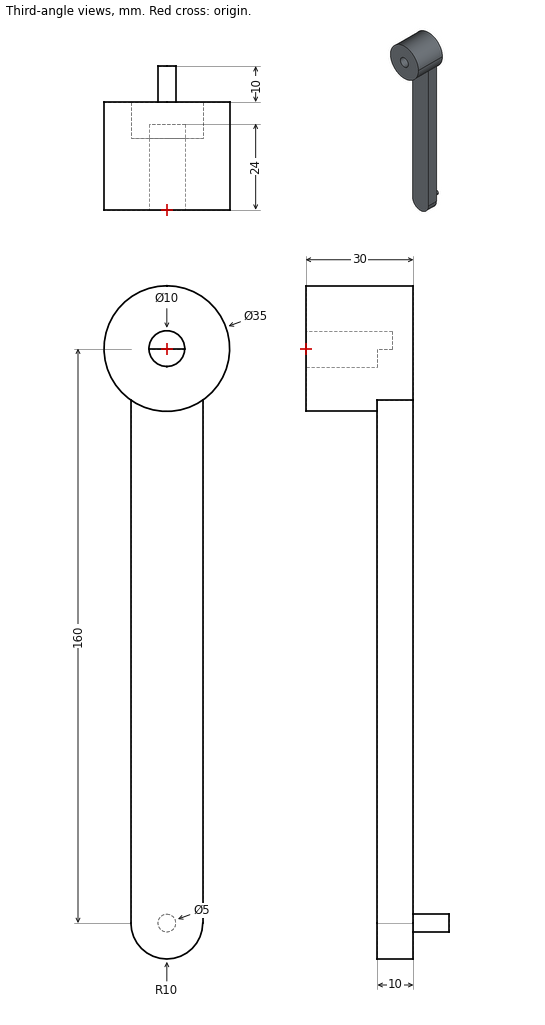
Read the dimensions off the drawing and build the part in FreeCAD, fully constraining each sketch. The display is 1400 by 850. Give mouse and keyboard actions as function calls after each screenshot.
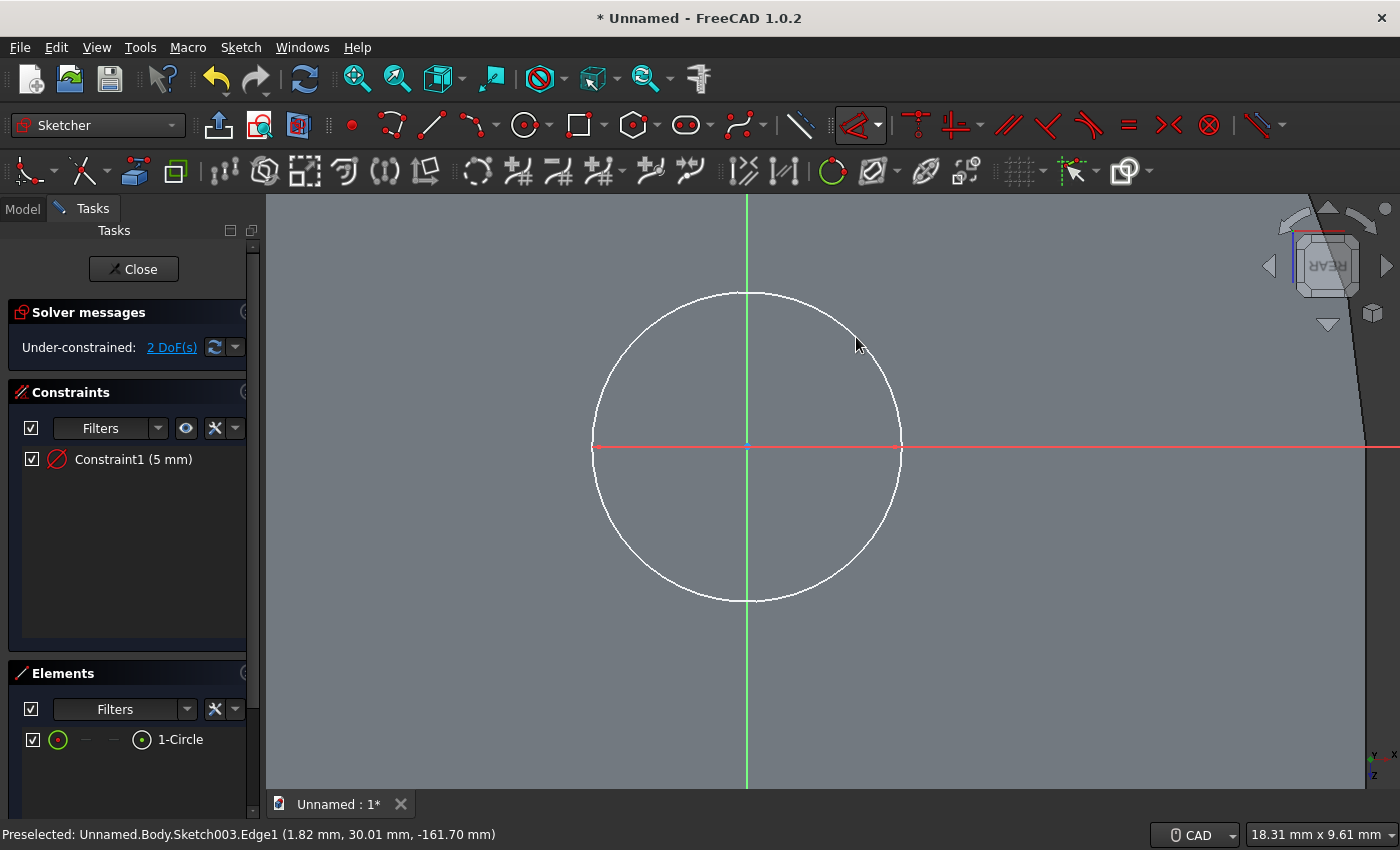
click(747, 447)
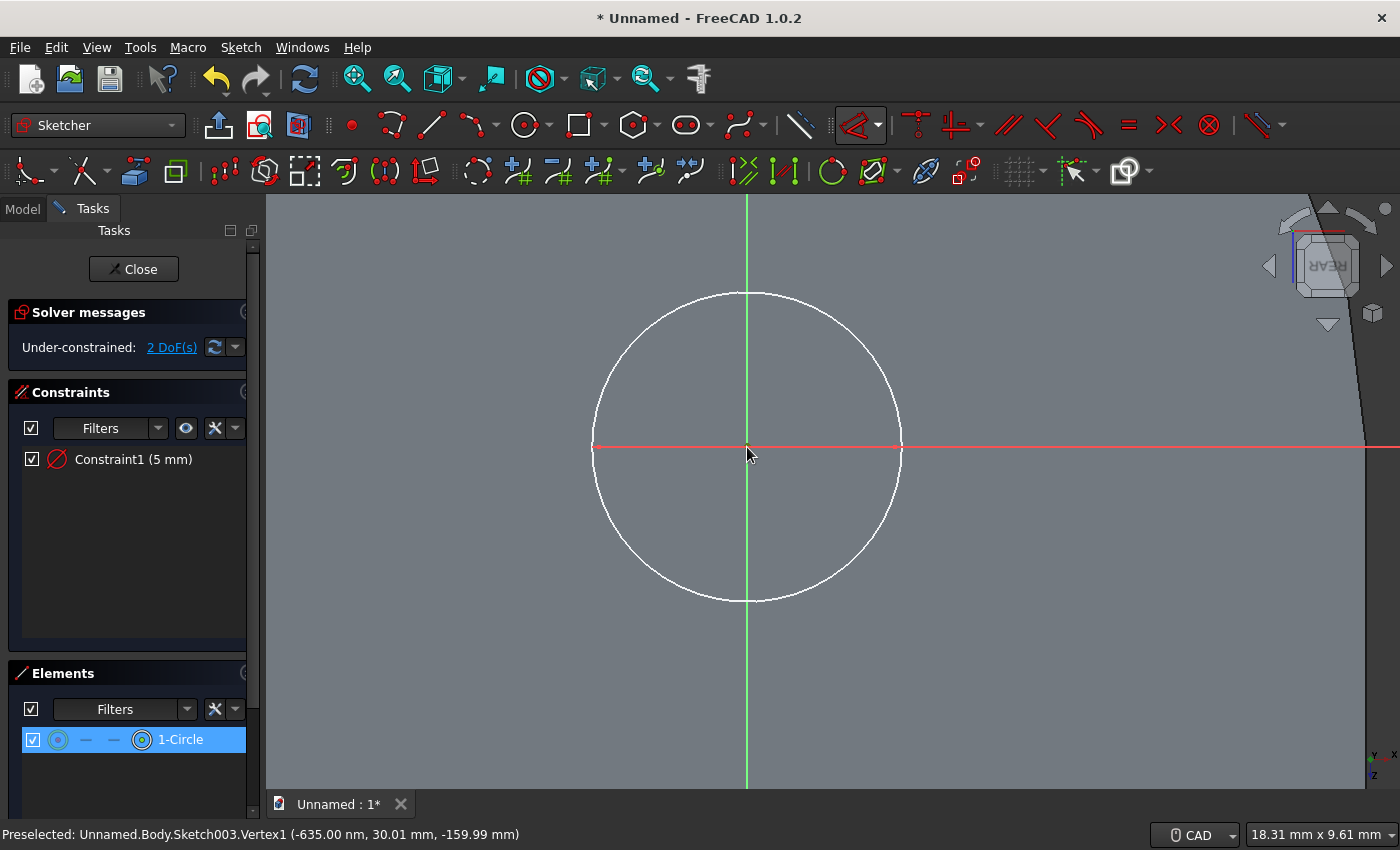
click(747, 722)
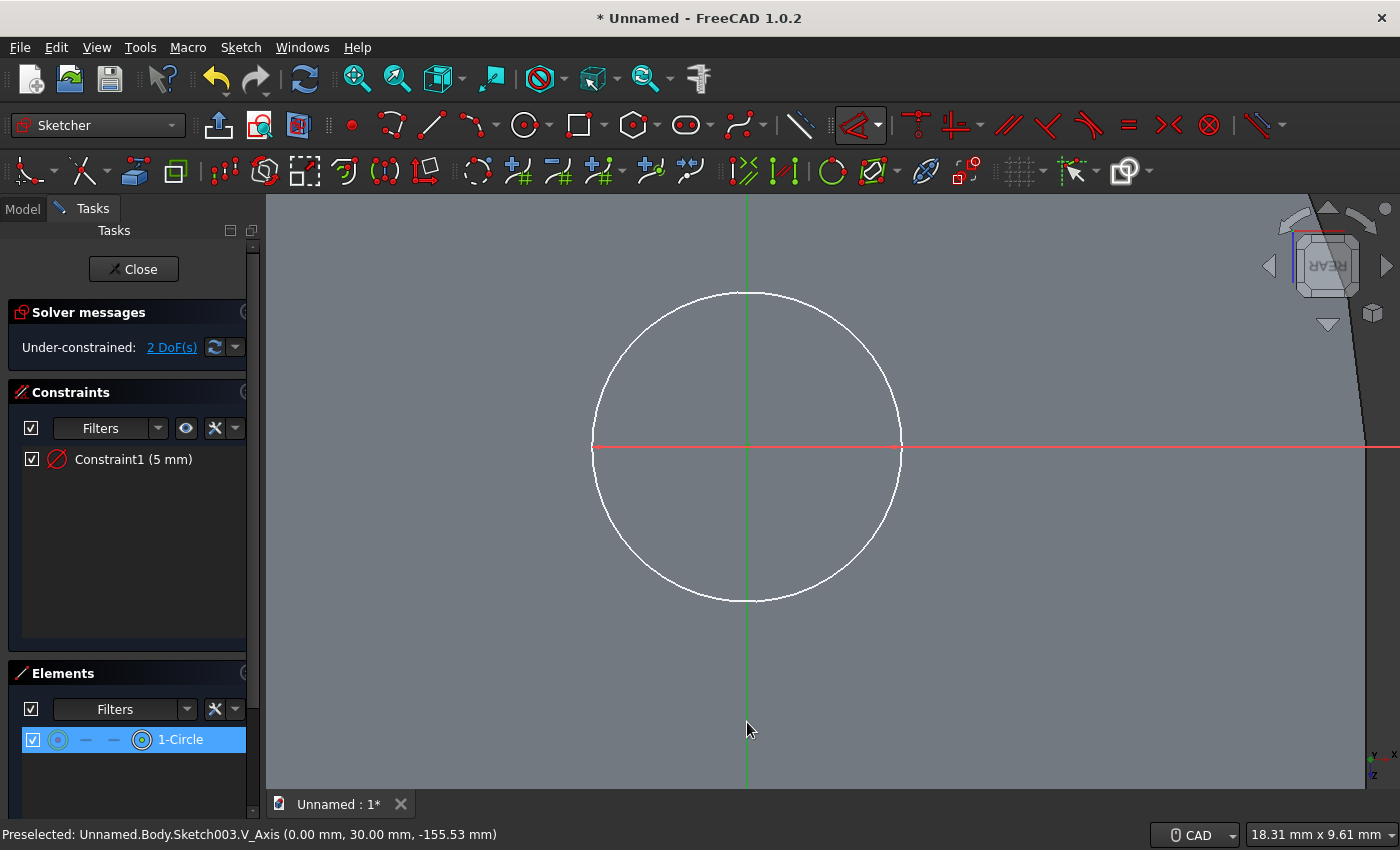
key(c)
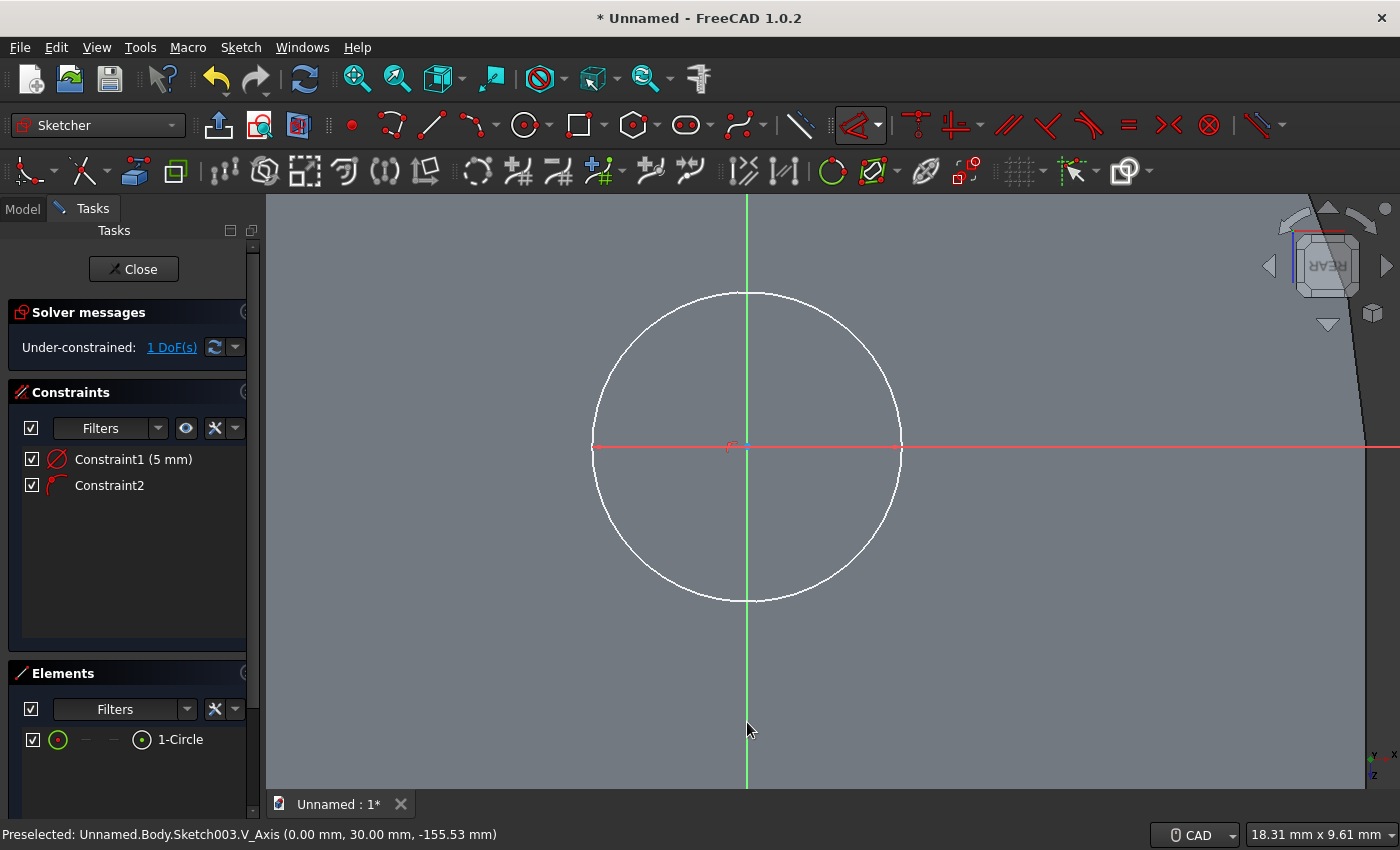
click(854, 126)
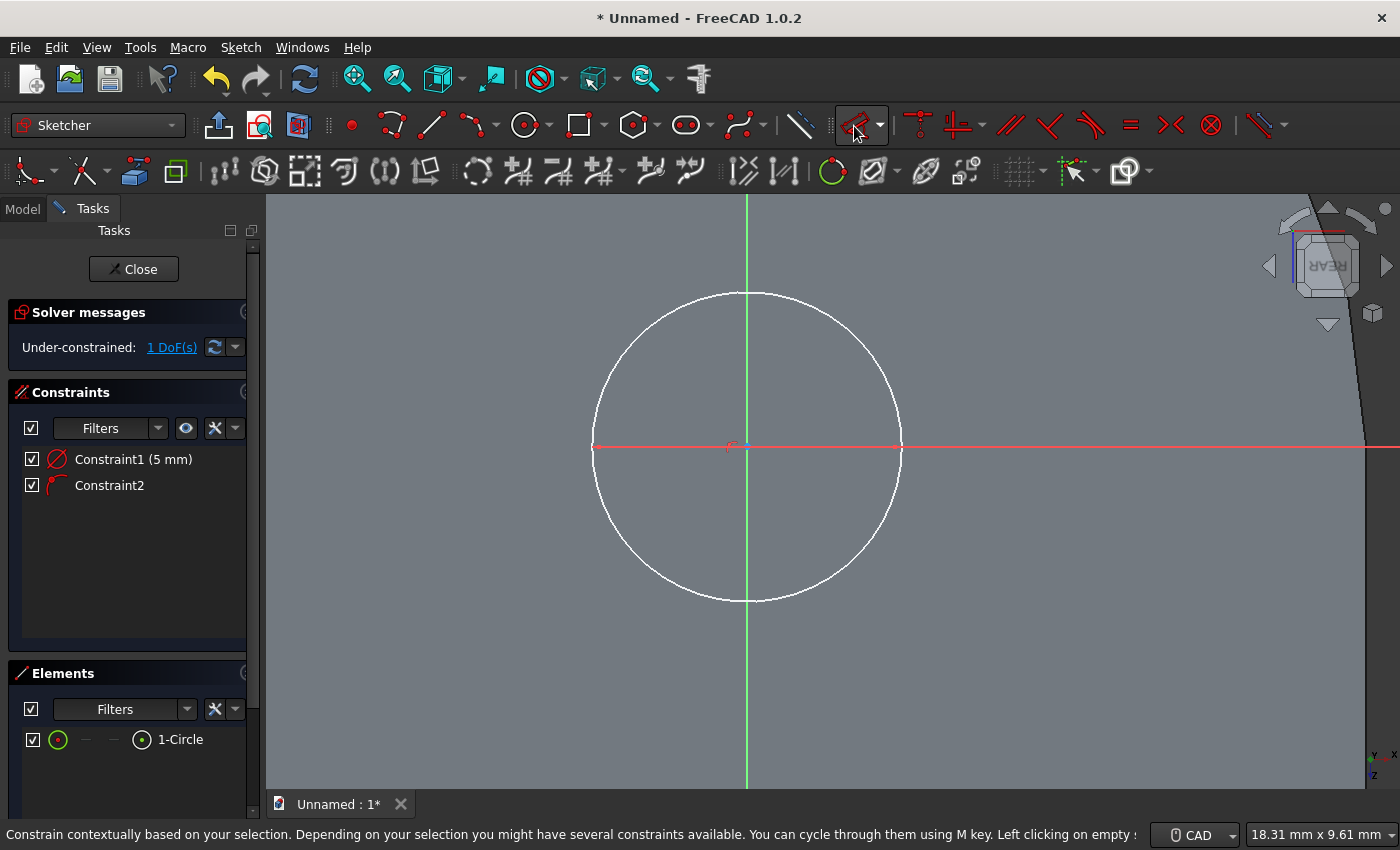
click(747, 447)
click(781, 532)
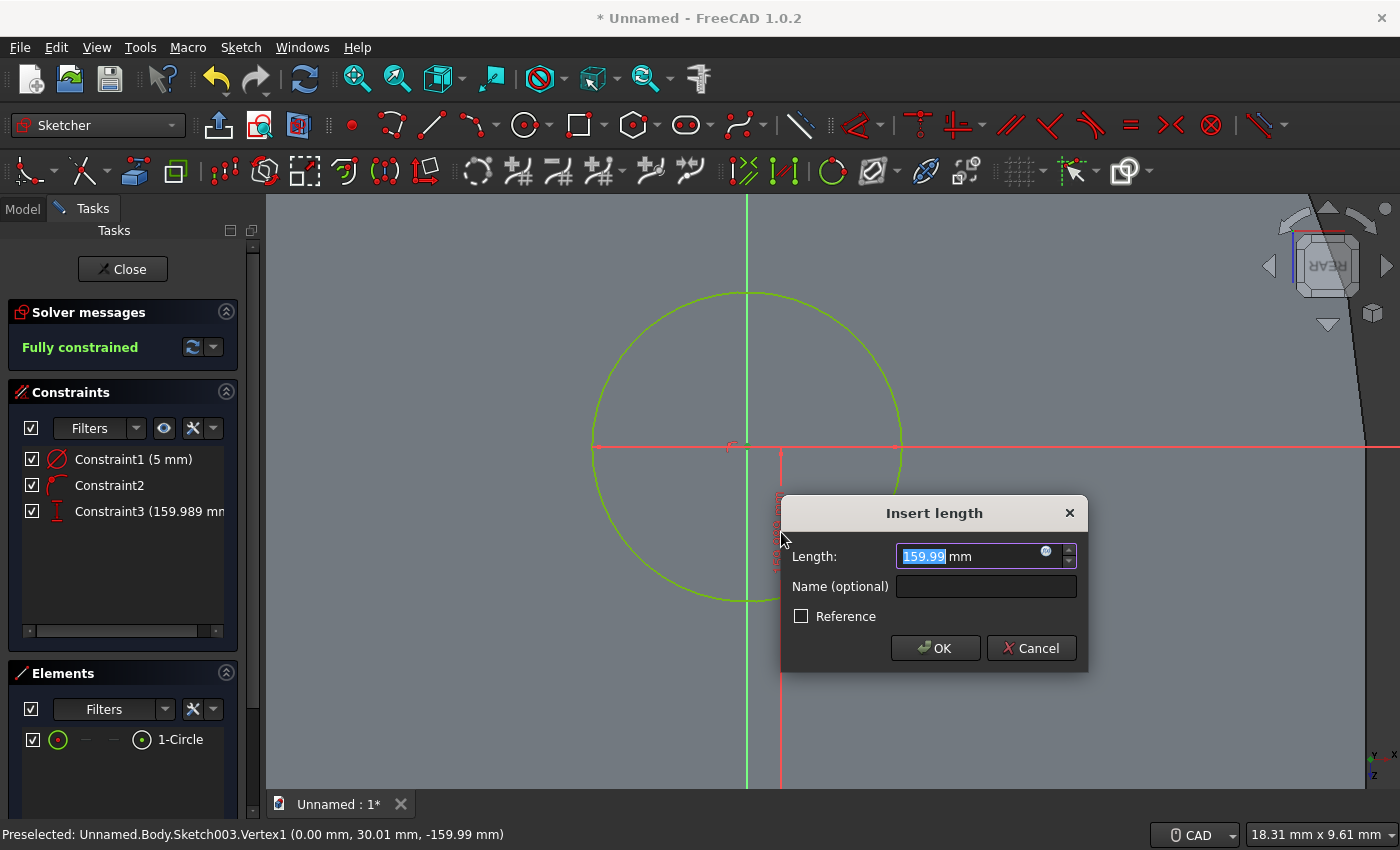
text(160)
key(Return)
key(Escape)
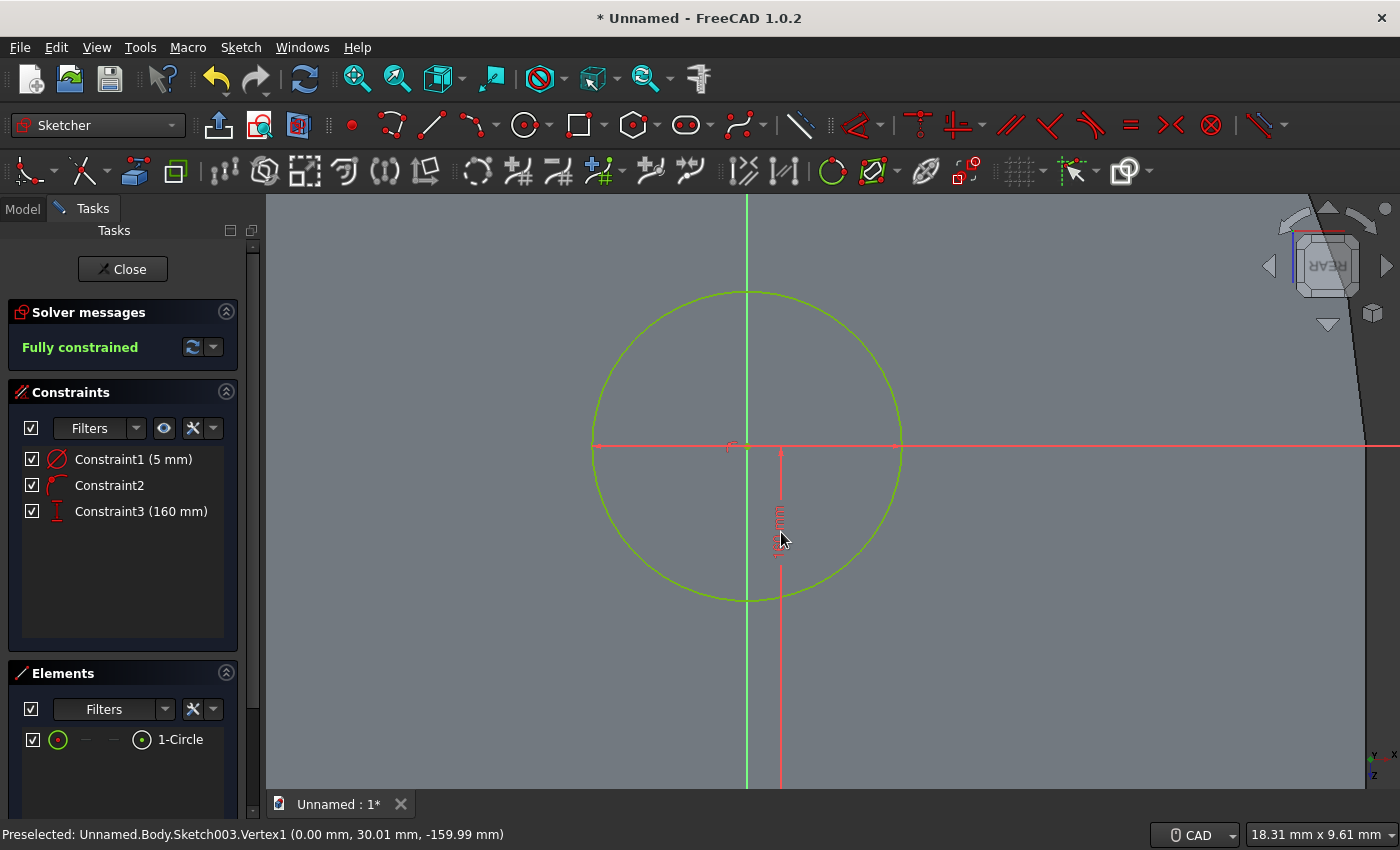
click(123, 269)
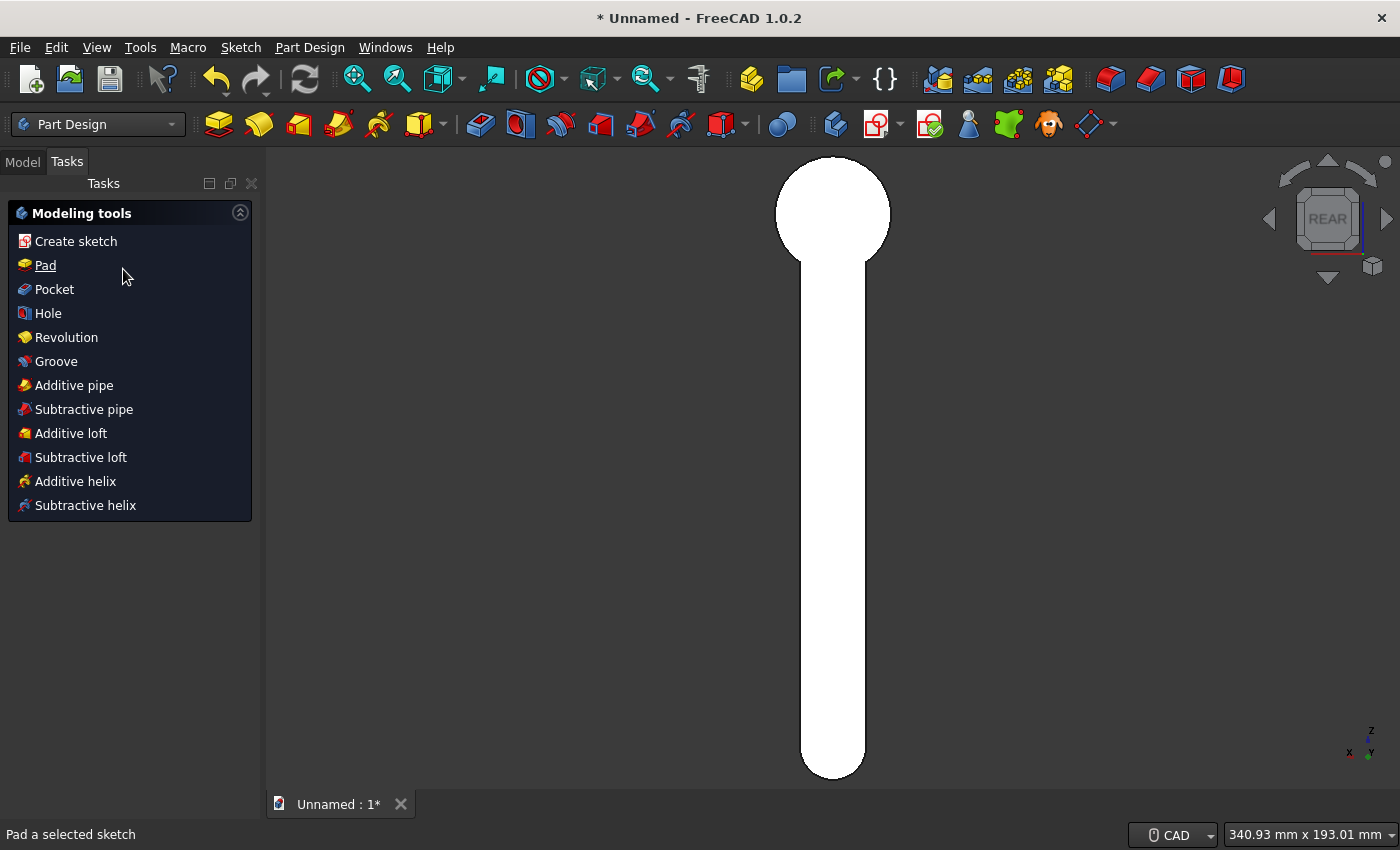
click(220, 124)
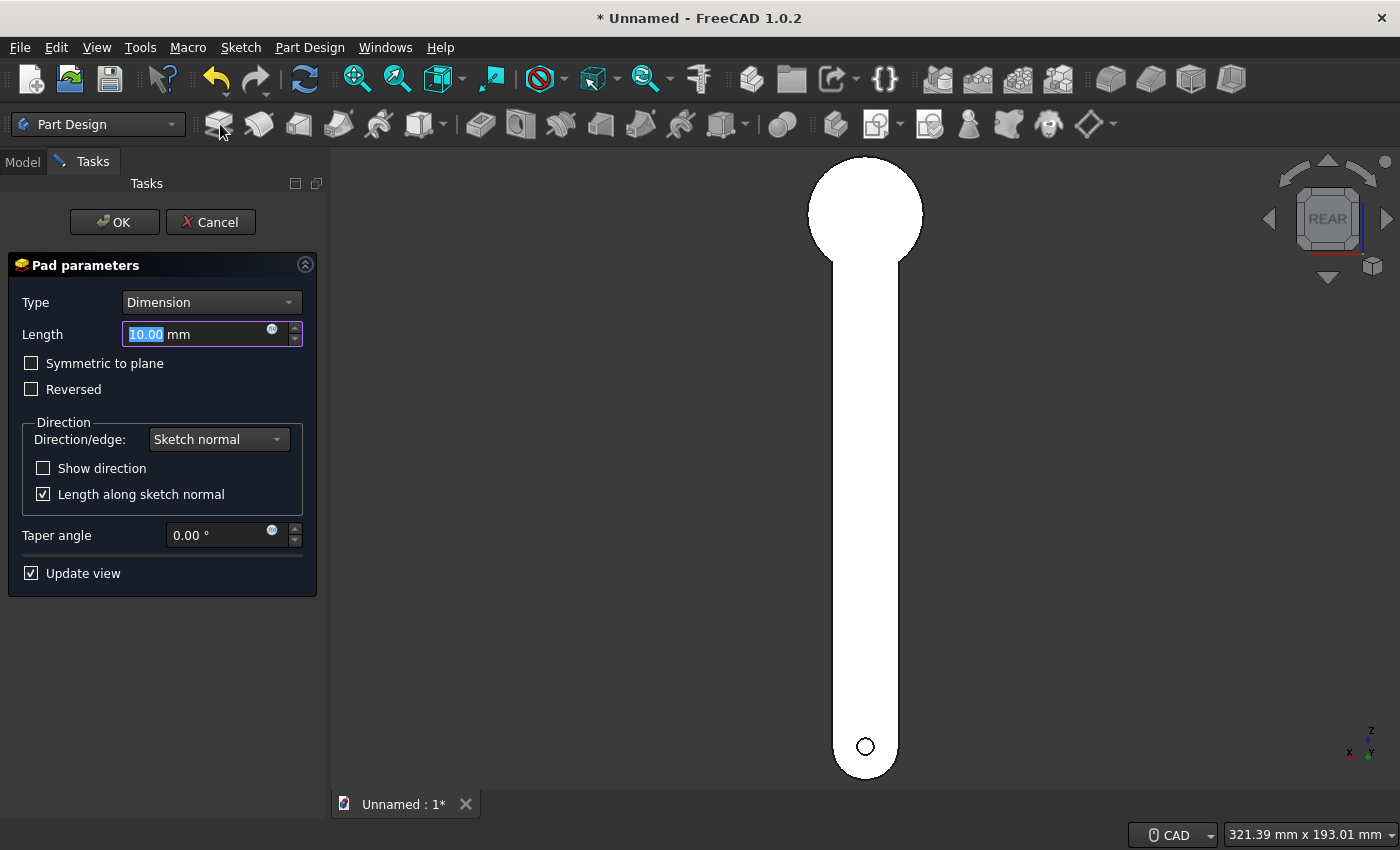
text(10)
key(Tab)